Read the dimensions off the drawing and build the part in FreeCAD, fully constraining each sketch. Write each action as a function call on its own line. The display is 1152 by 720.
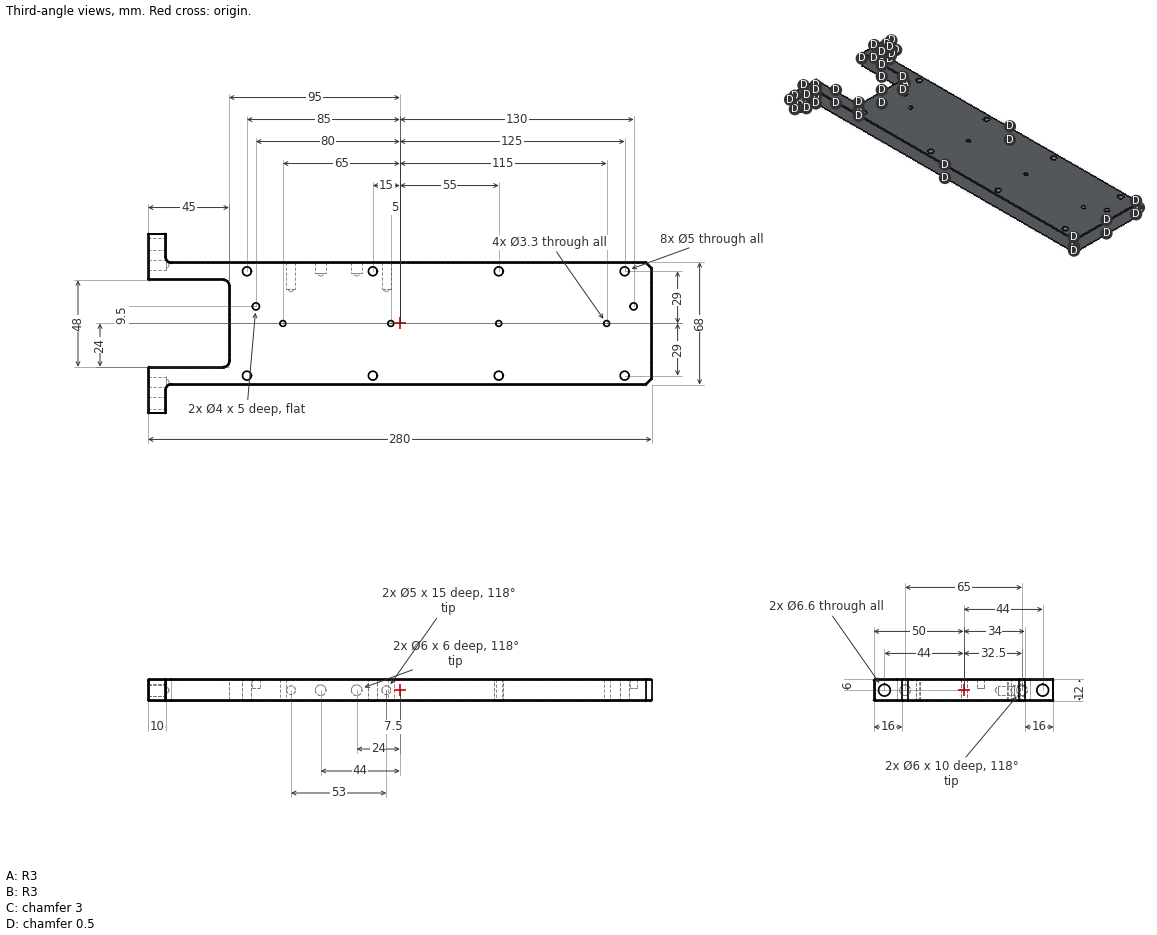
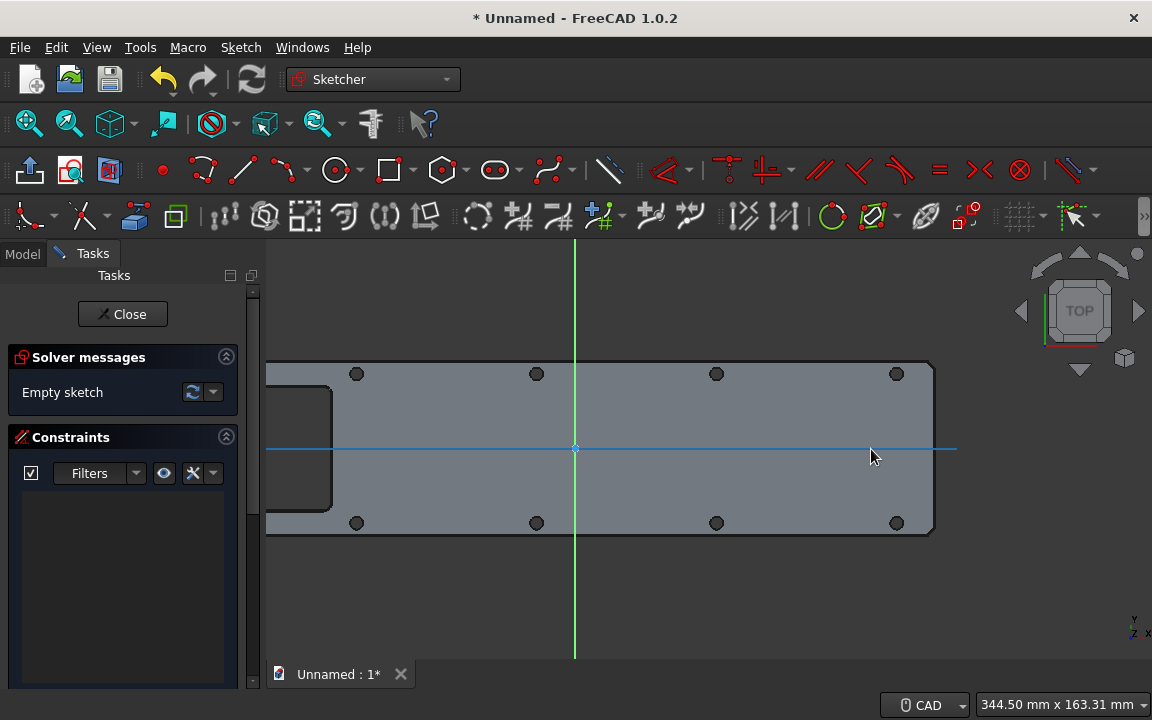
click(336, 170)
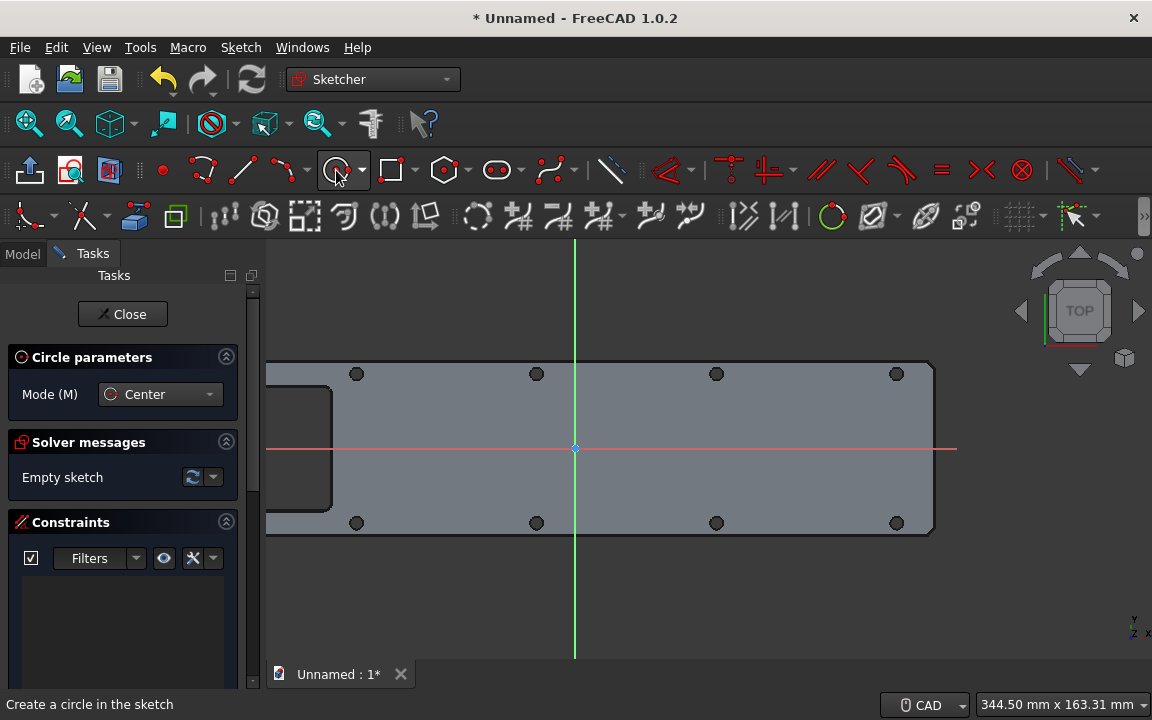
scroll(871, 449, up, 9)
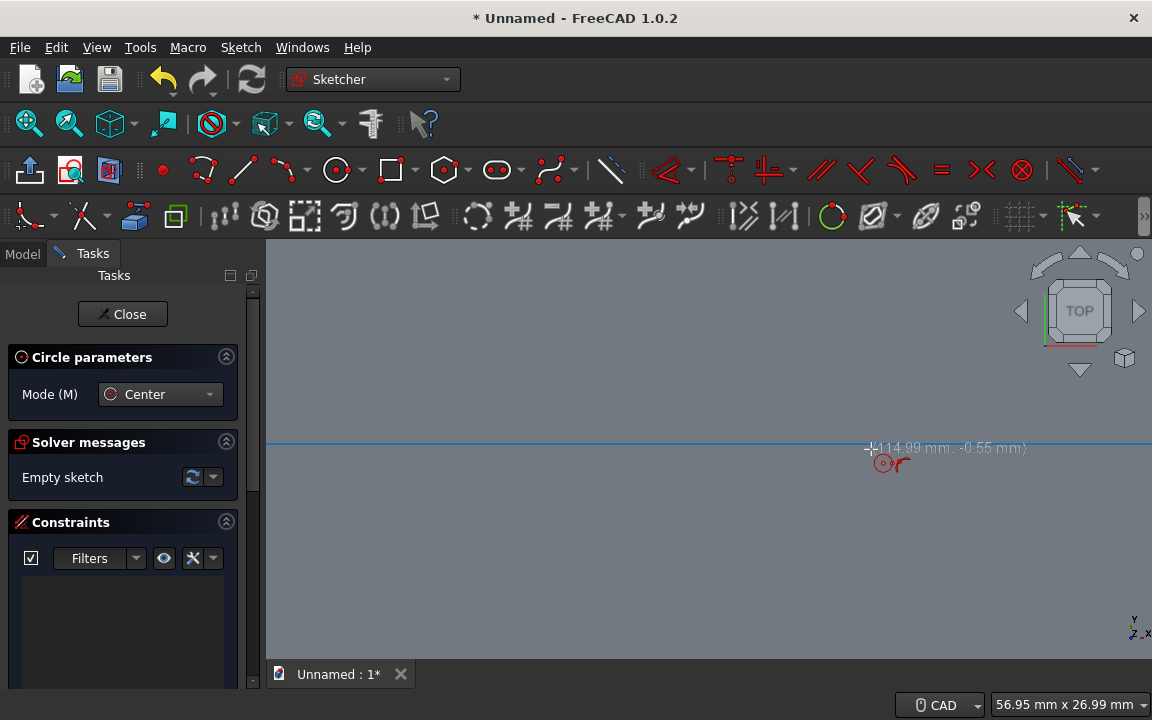
scroll(873, 450, down, 9)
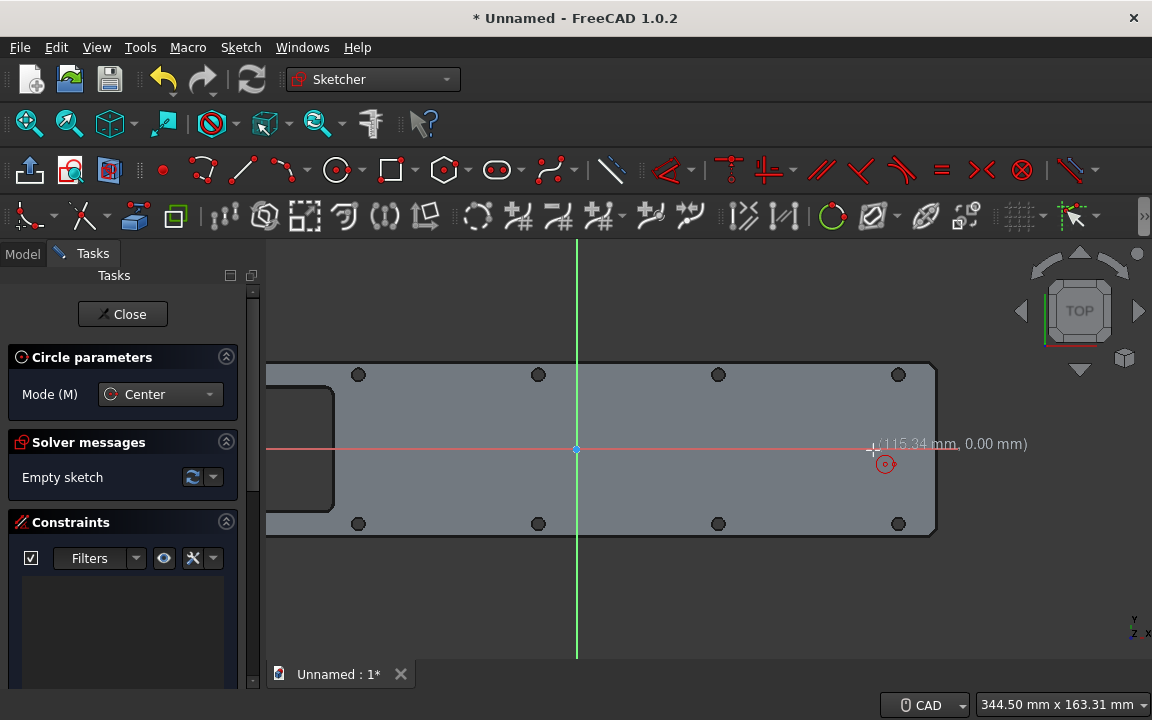
click(873, 449)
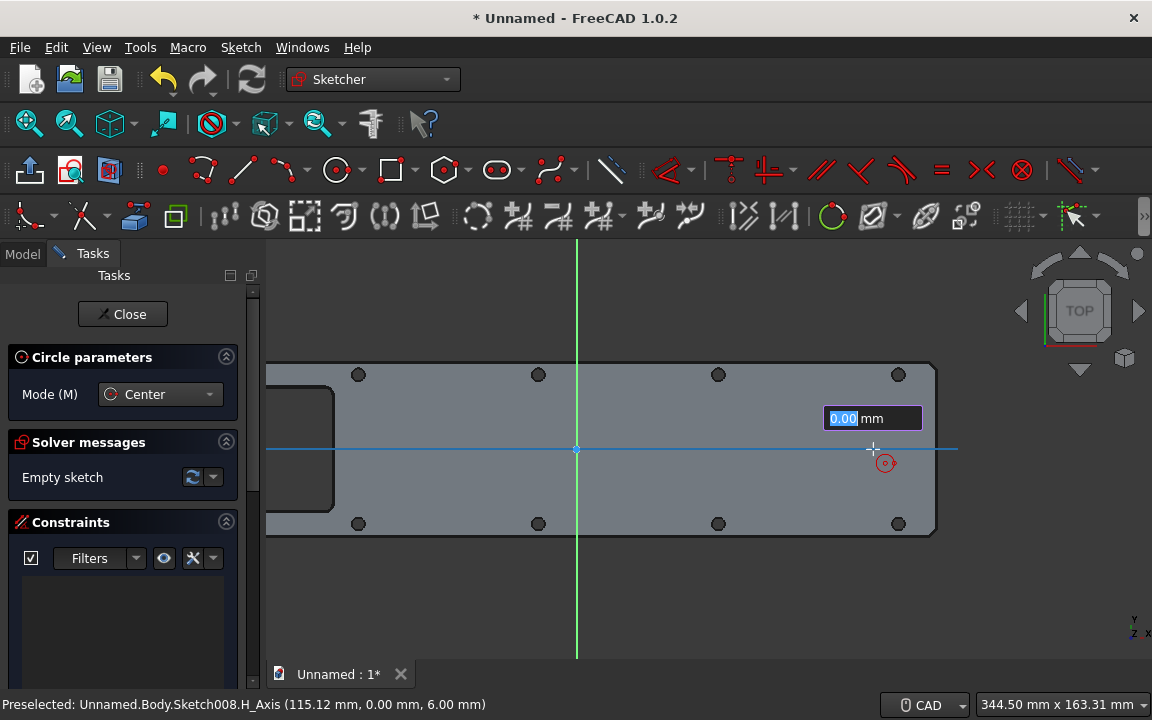
scroll(871, 453, up, 7)
move(870, 453)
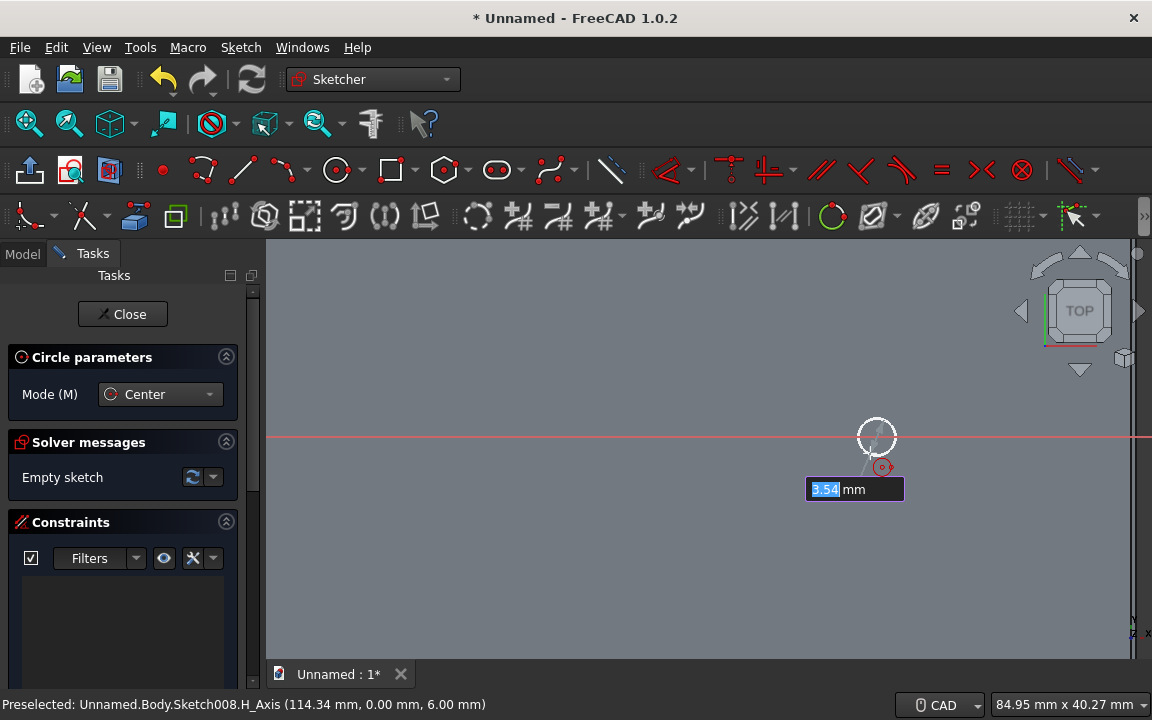
text(3.3)
key(Return)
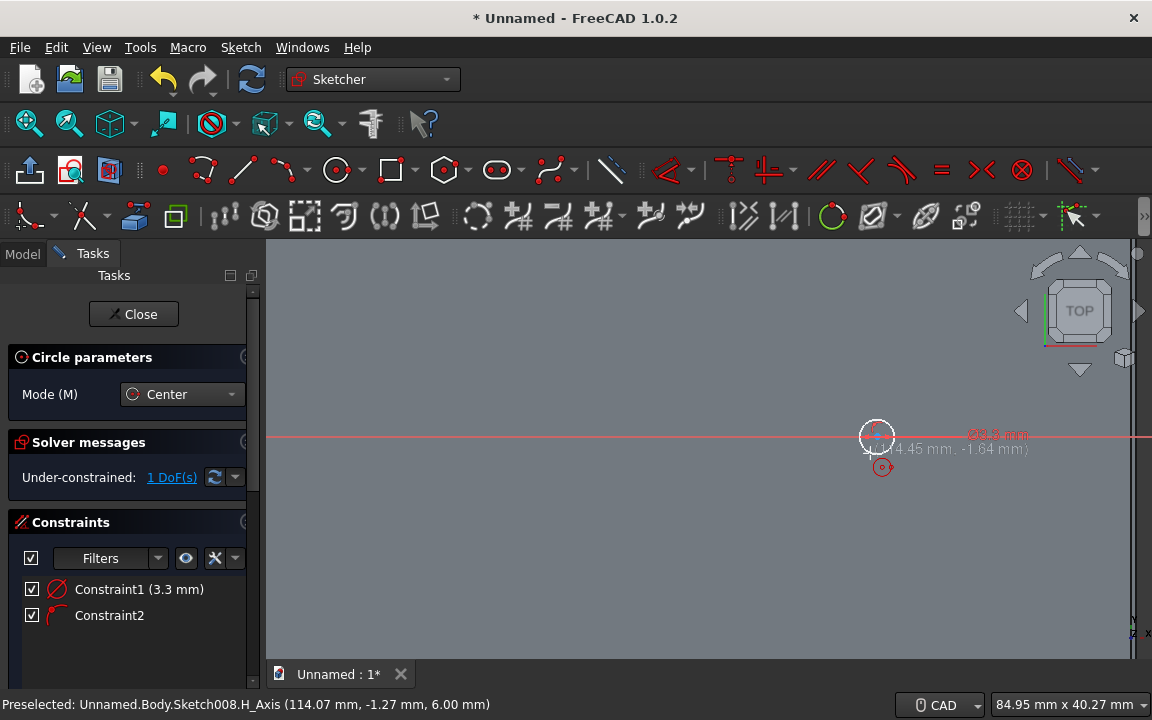
scroll(871, 453, down, 7)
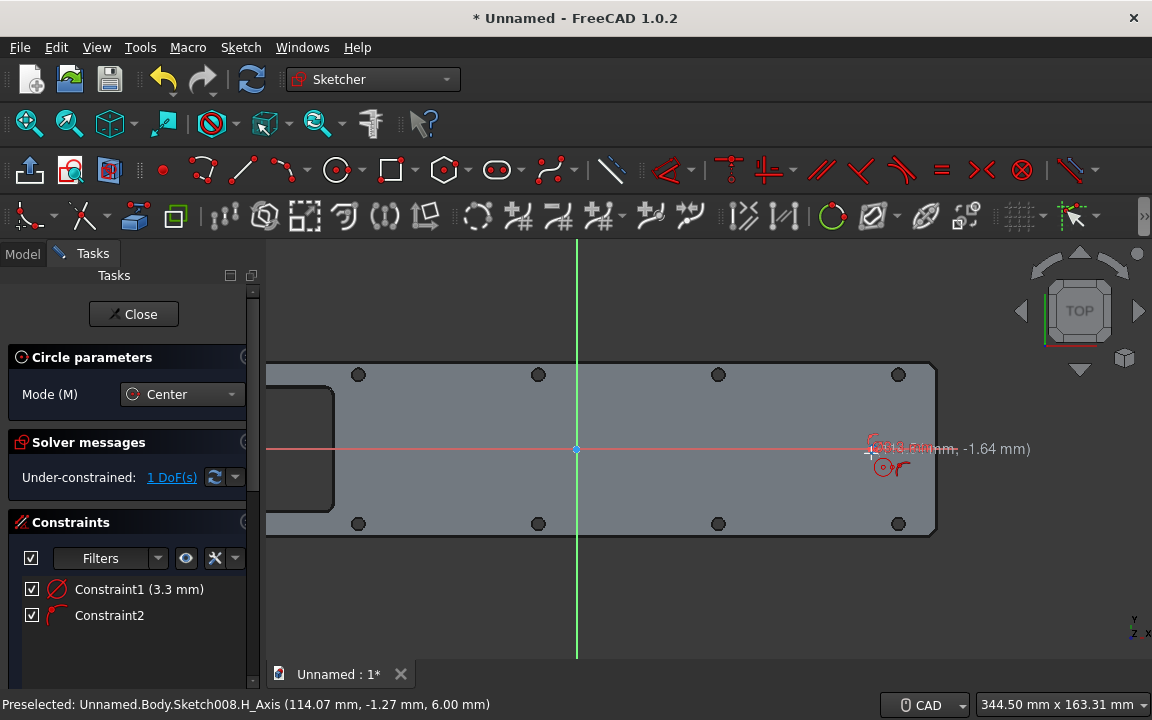
scroll(718, 449, up, 9)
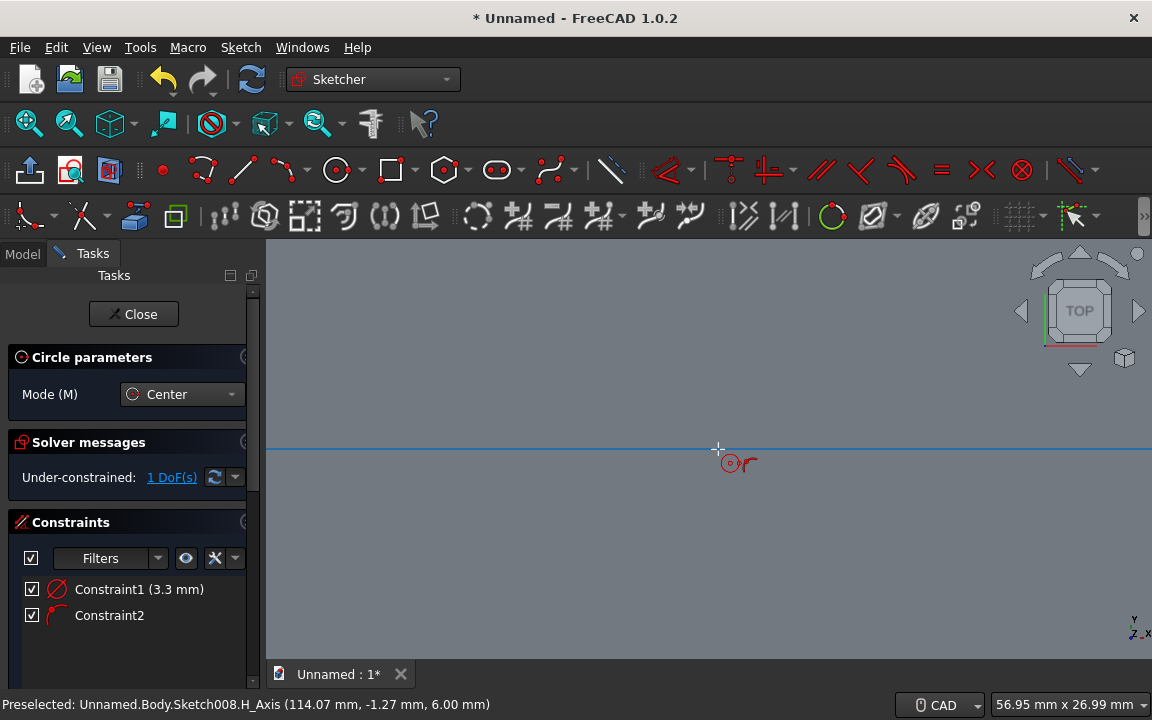
scroll(718, 449, down, 9)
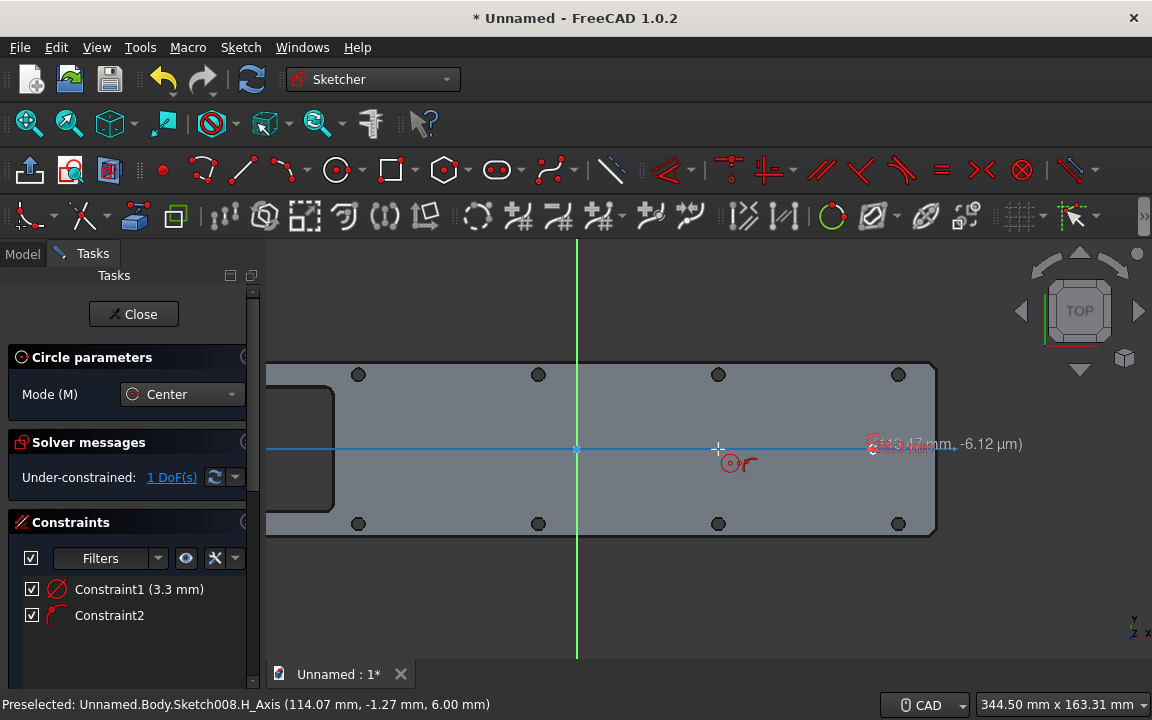
click(718, 449)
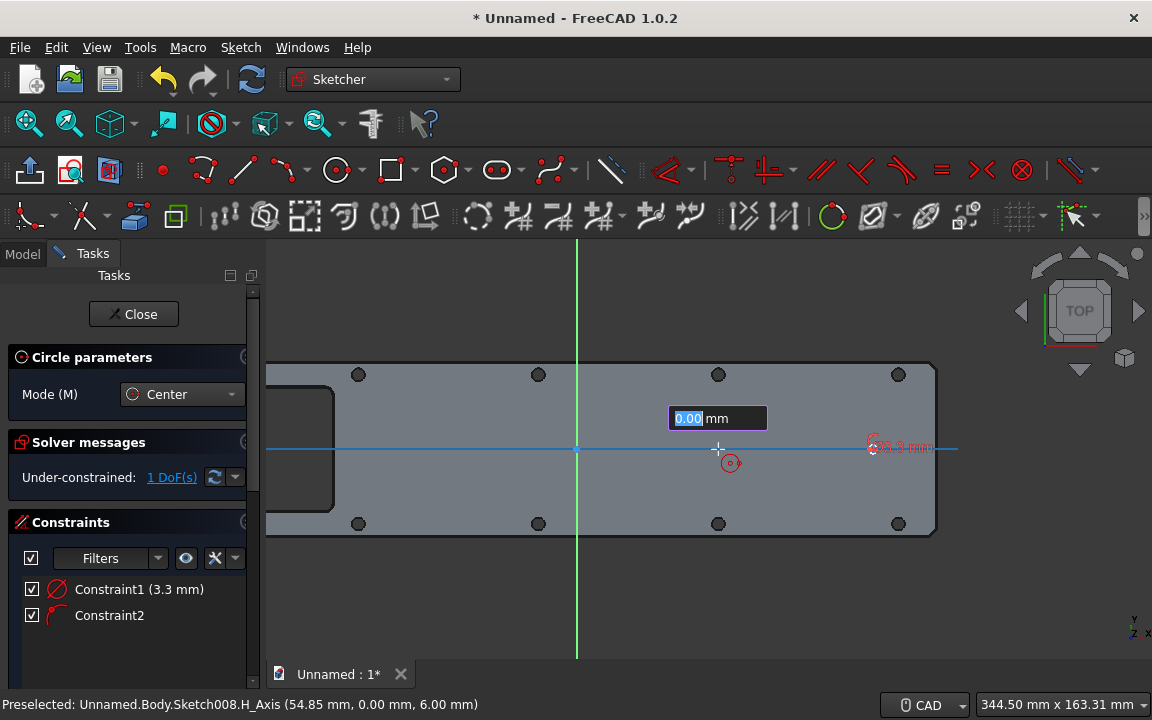
scroll(717, 453, up, 7)
move(715, 453)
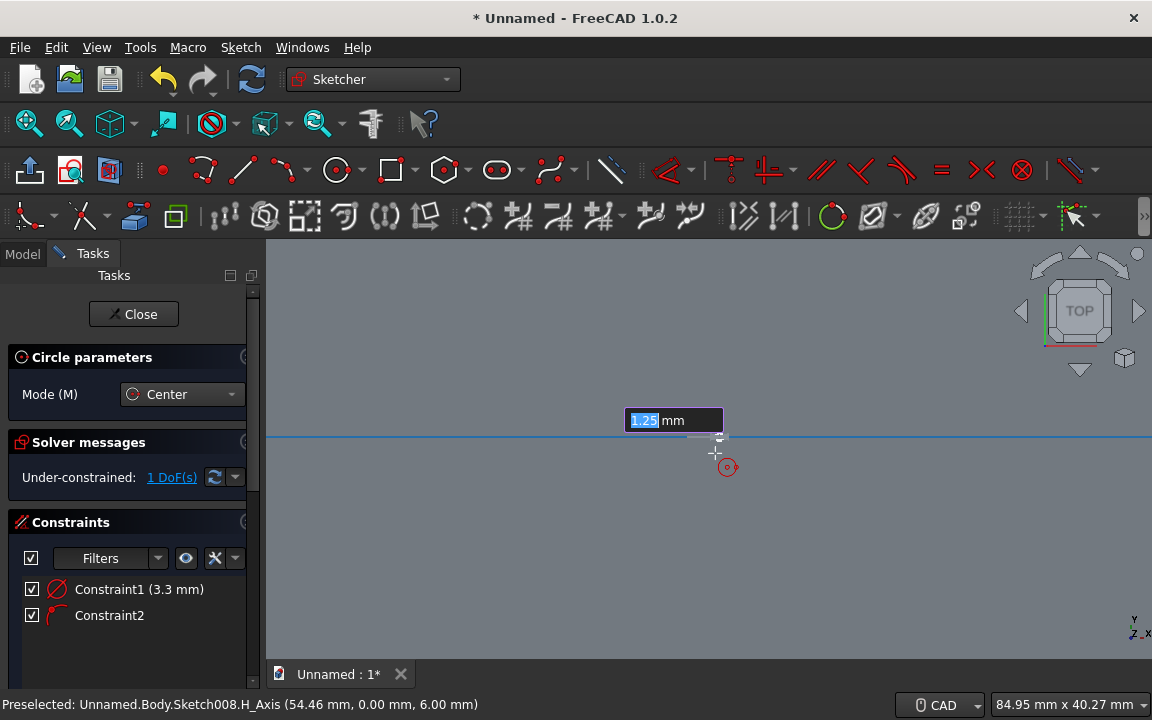
text(3.3)
key(Return)